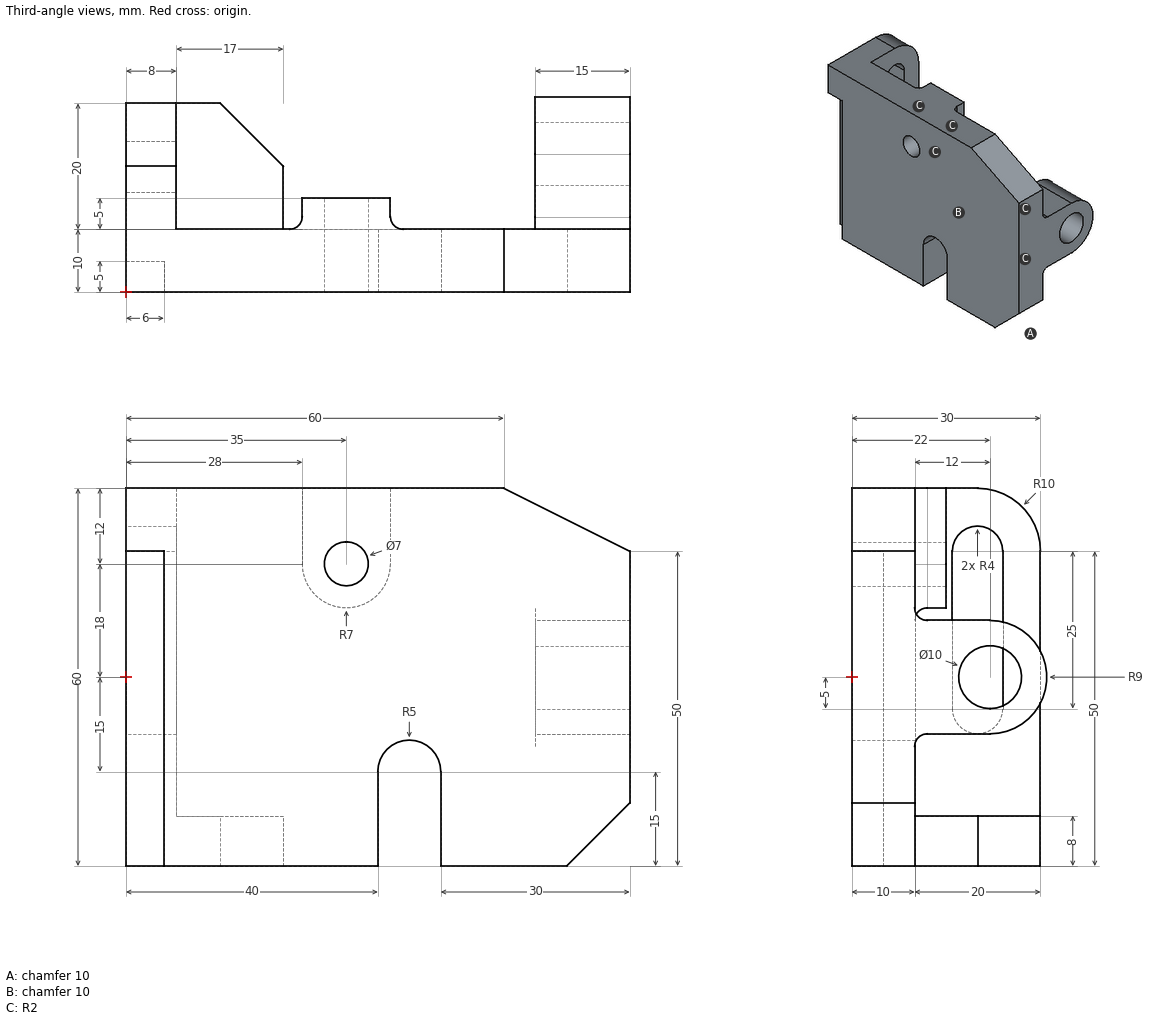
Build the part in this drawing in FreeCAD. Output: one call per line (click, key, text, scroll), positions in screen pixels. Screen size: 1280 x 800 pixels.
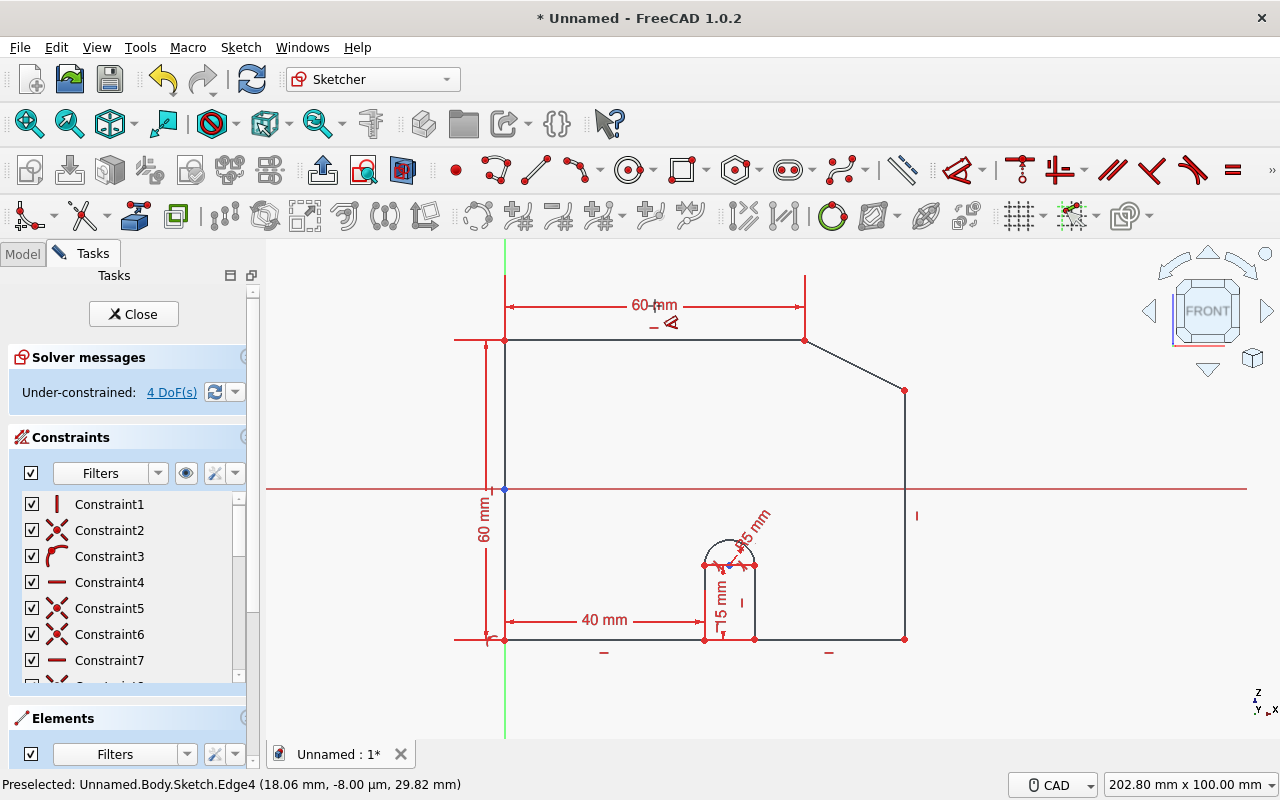
click(905, 465)
click(939, 515)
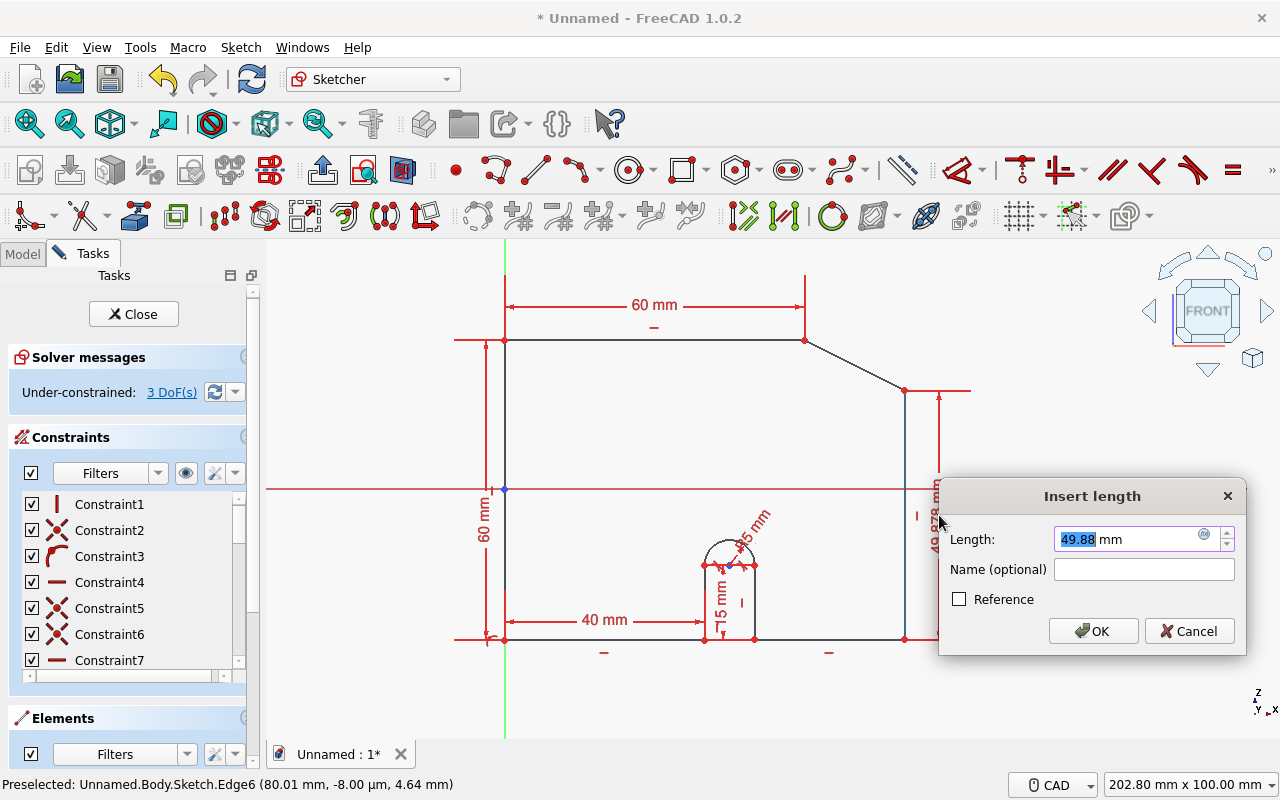
text(50)
key(Return)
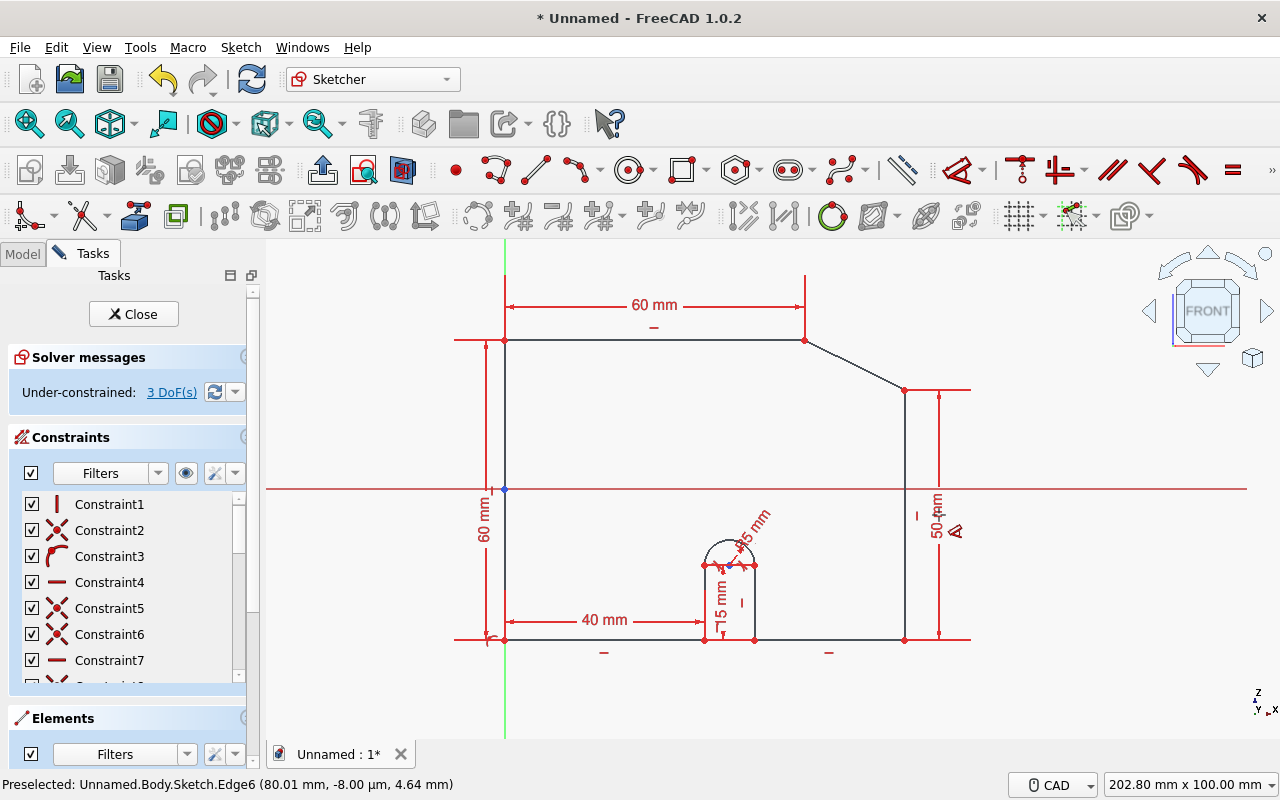
click(860, 640)
click(830, 674)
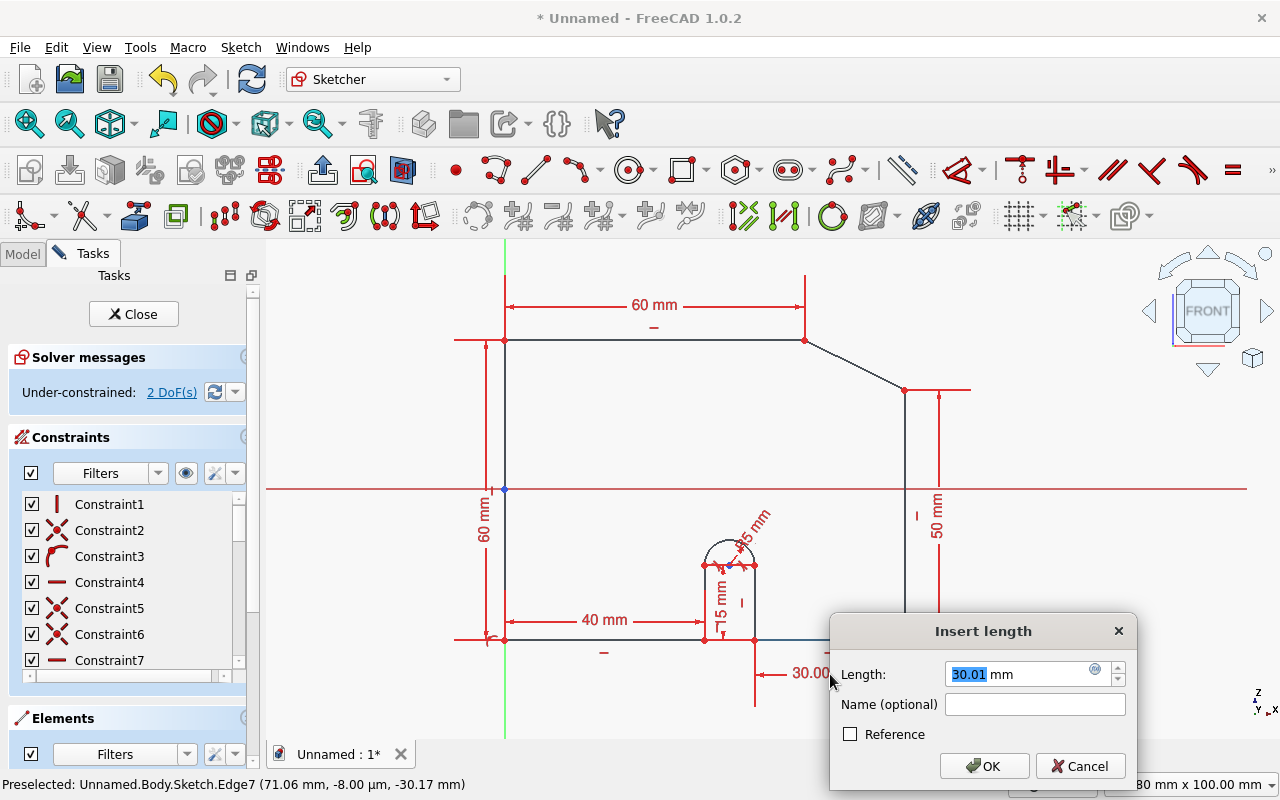
text(30)
key(Return)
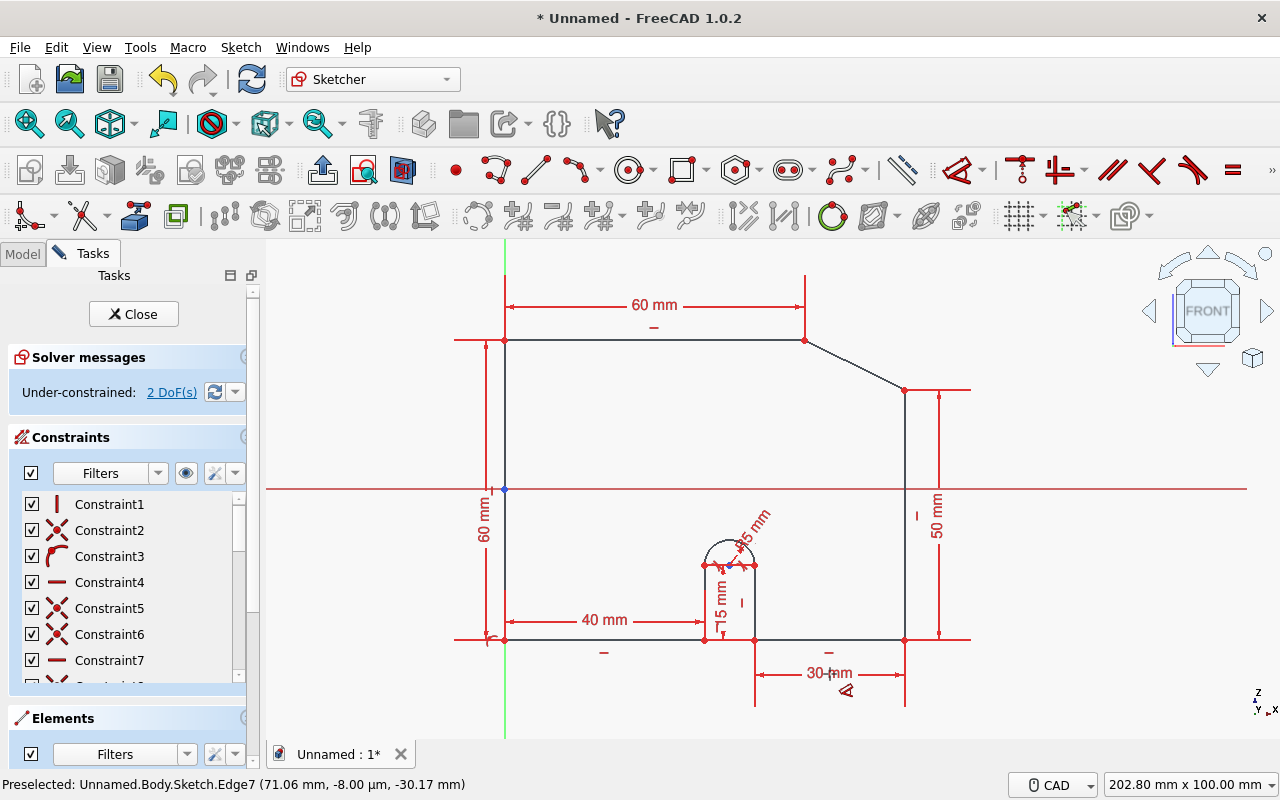
click(755, 618)
click(789, 576)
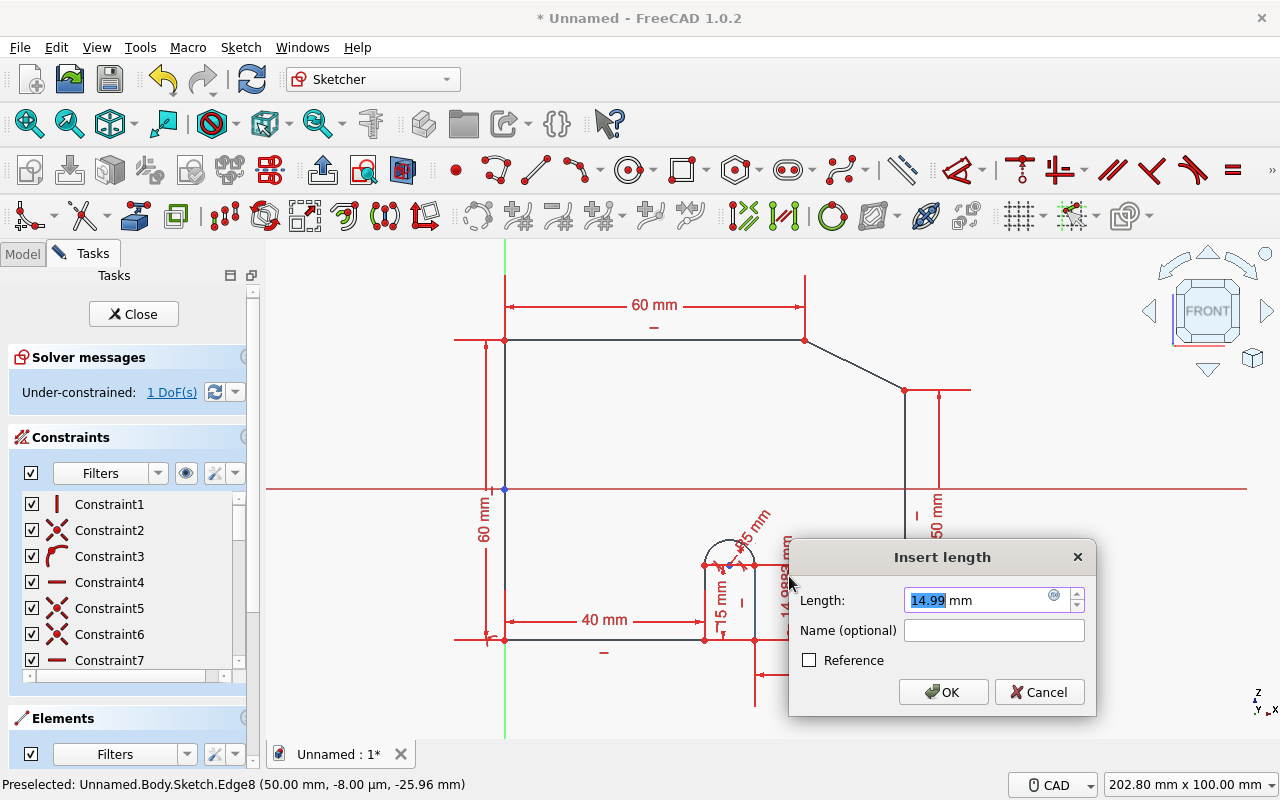
text(15)
key(Return)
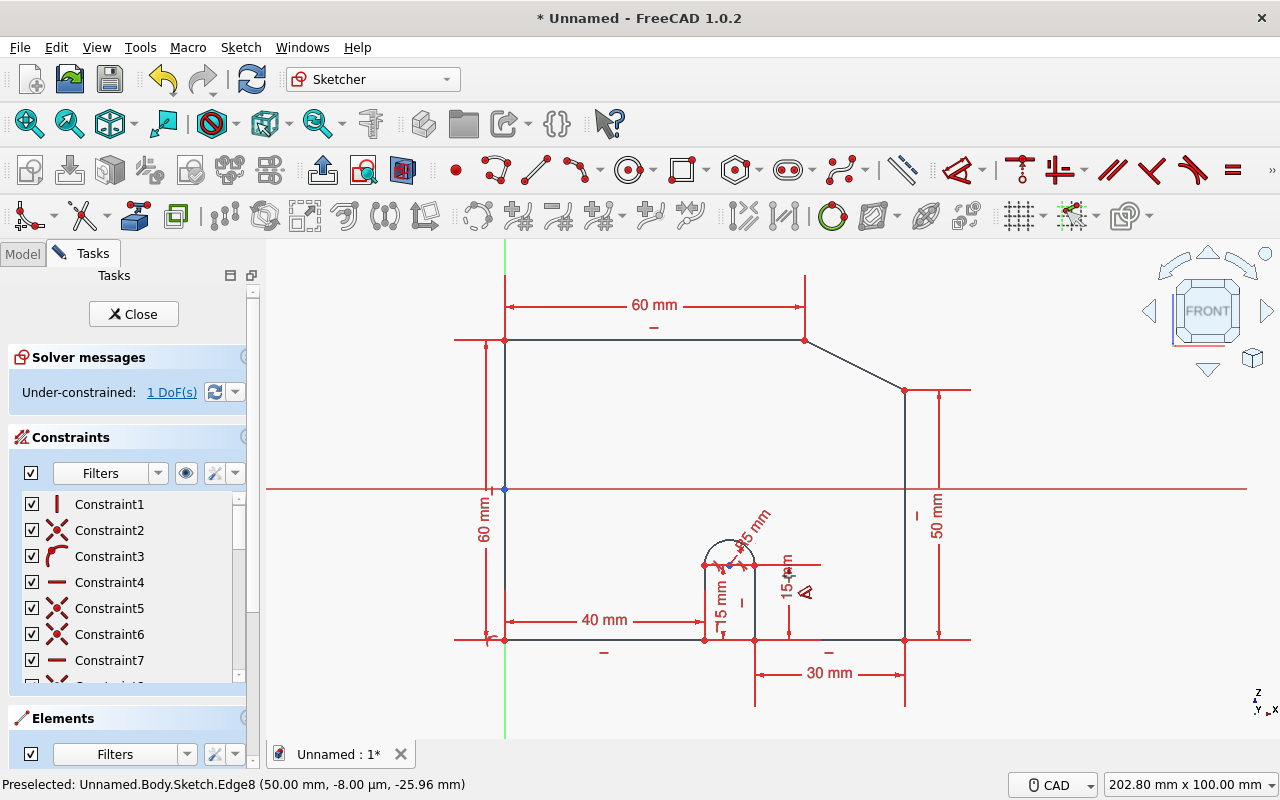
click(705, 565)
click(471, 545)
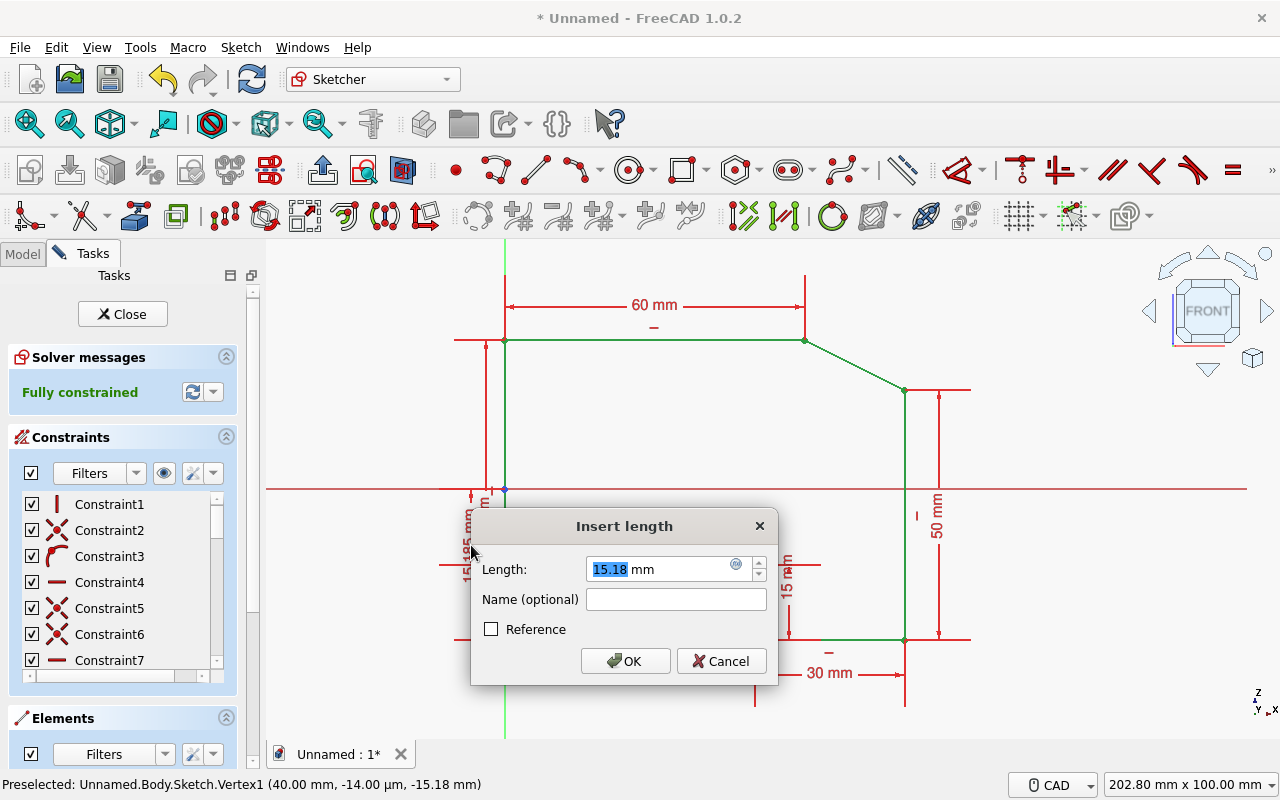
text(15)
key(Return)
key(Escape)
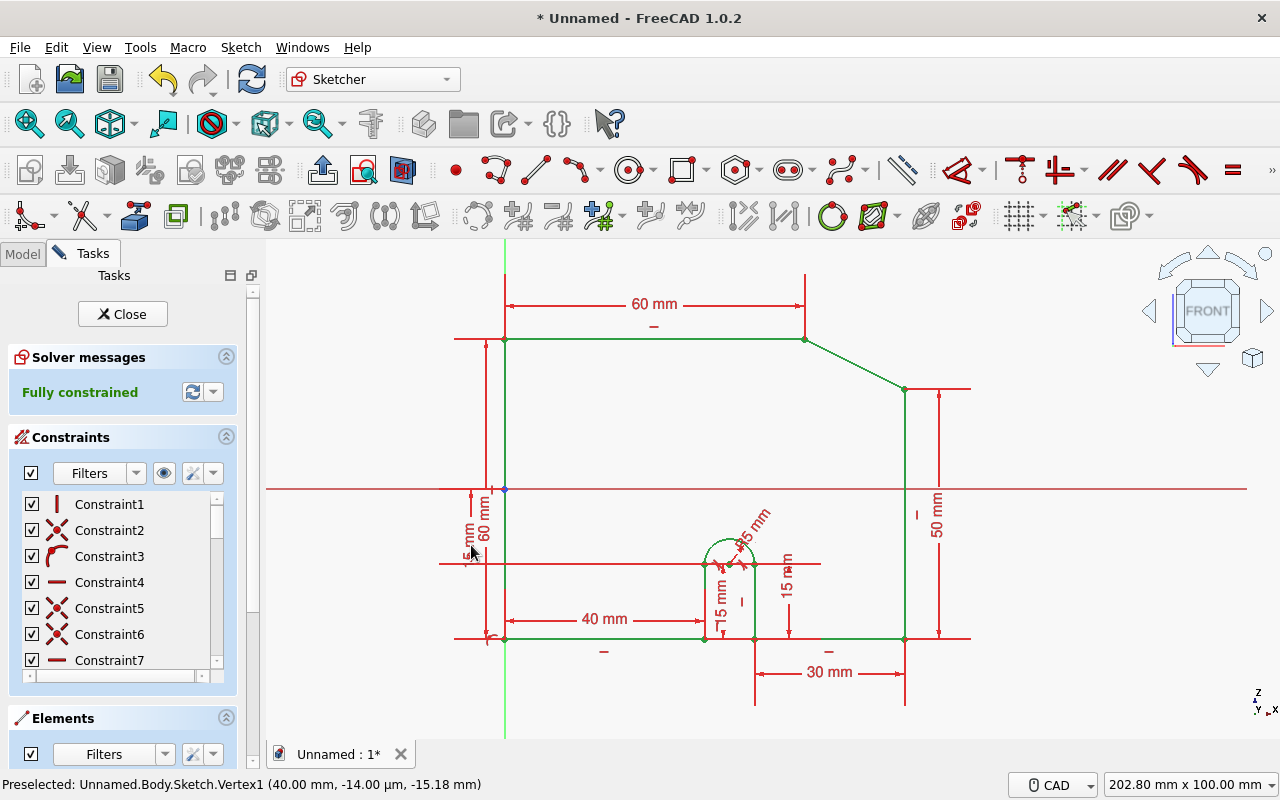
click(123, 314)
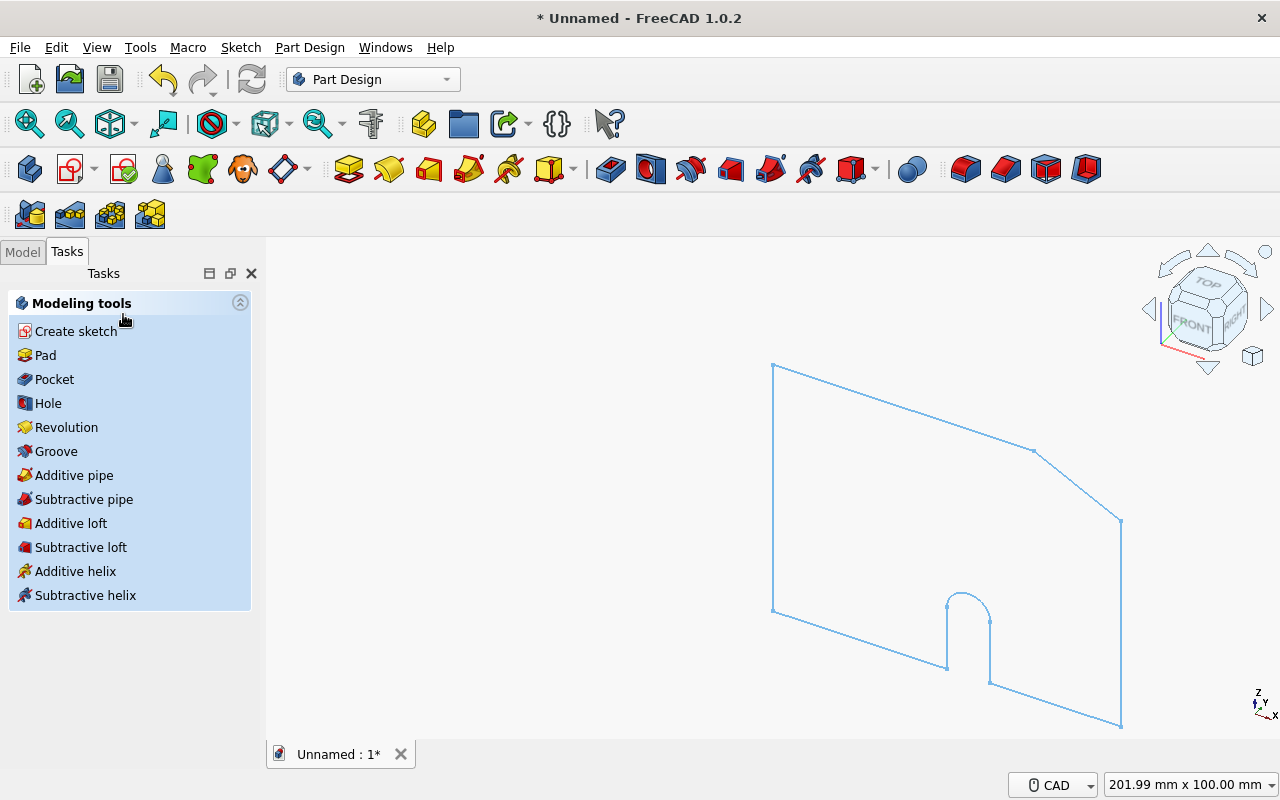
click(350, 170)